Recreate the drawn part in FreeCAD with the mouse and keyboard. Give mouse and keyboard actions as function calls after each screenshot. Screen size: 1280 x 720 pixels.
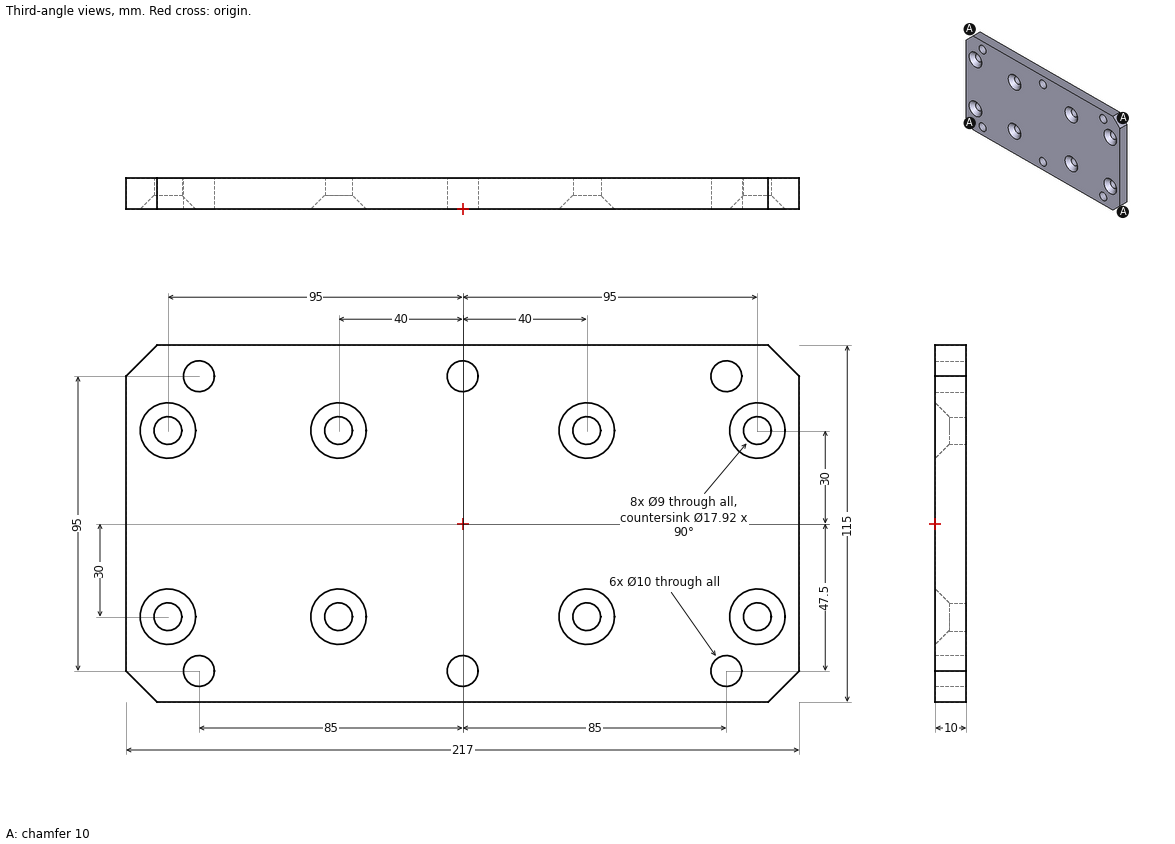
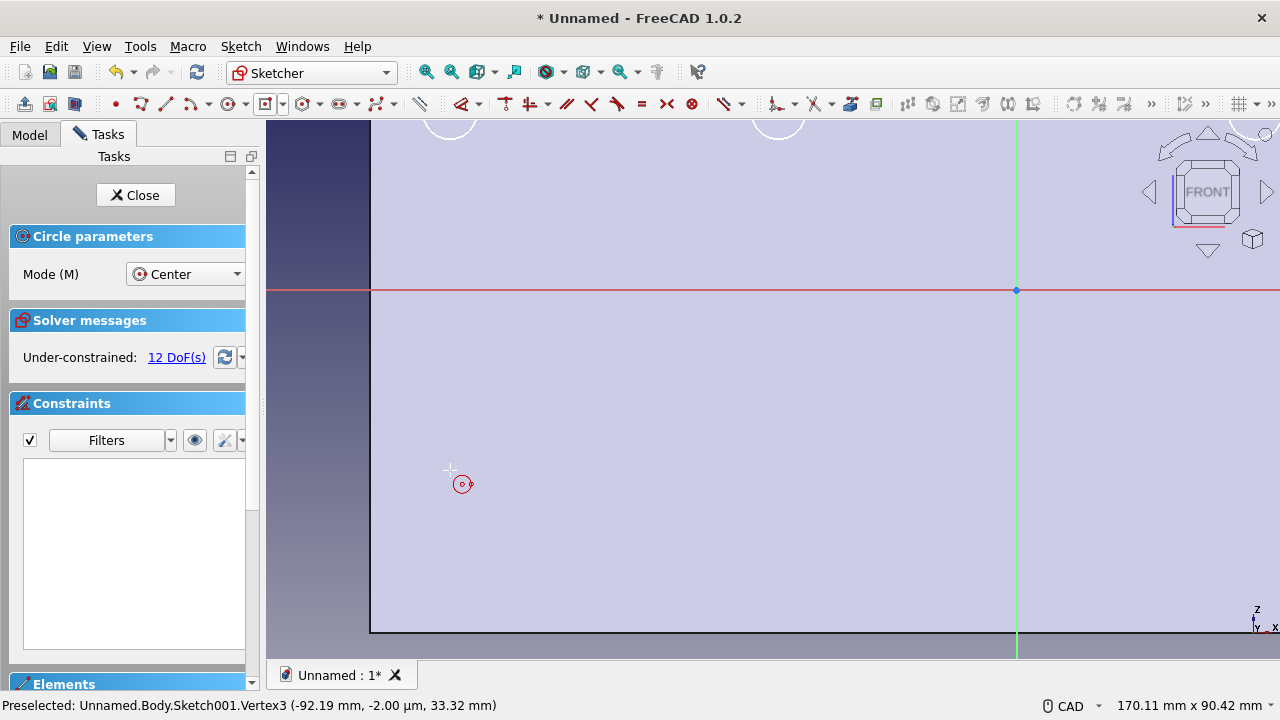
click(450, 469)
click(469, 450)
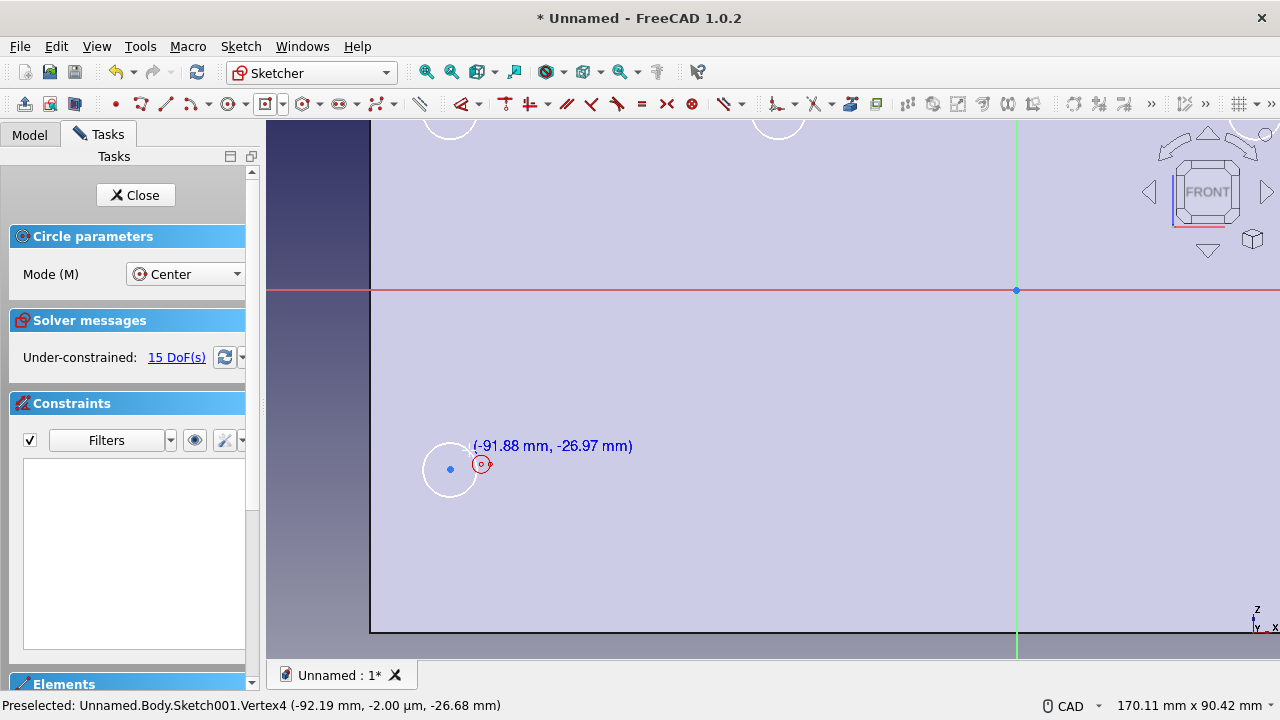
click(778, 469)
click(797, 450)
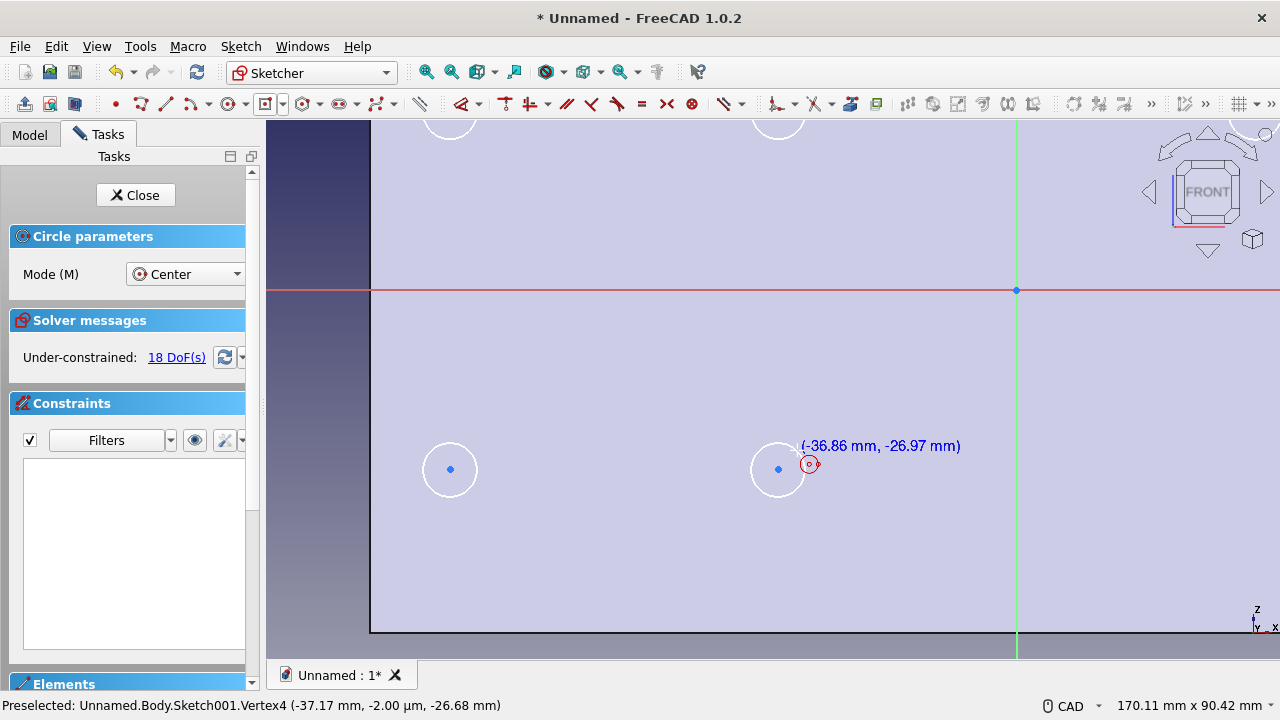
scroll(450, 471, down, 4)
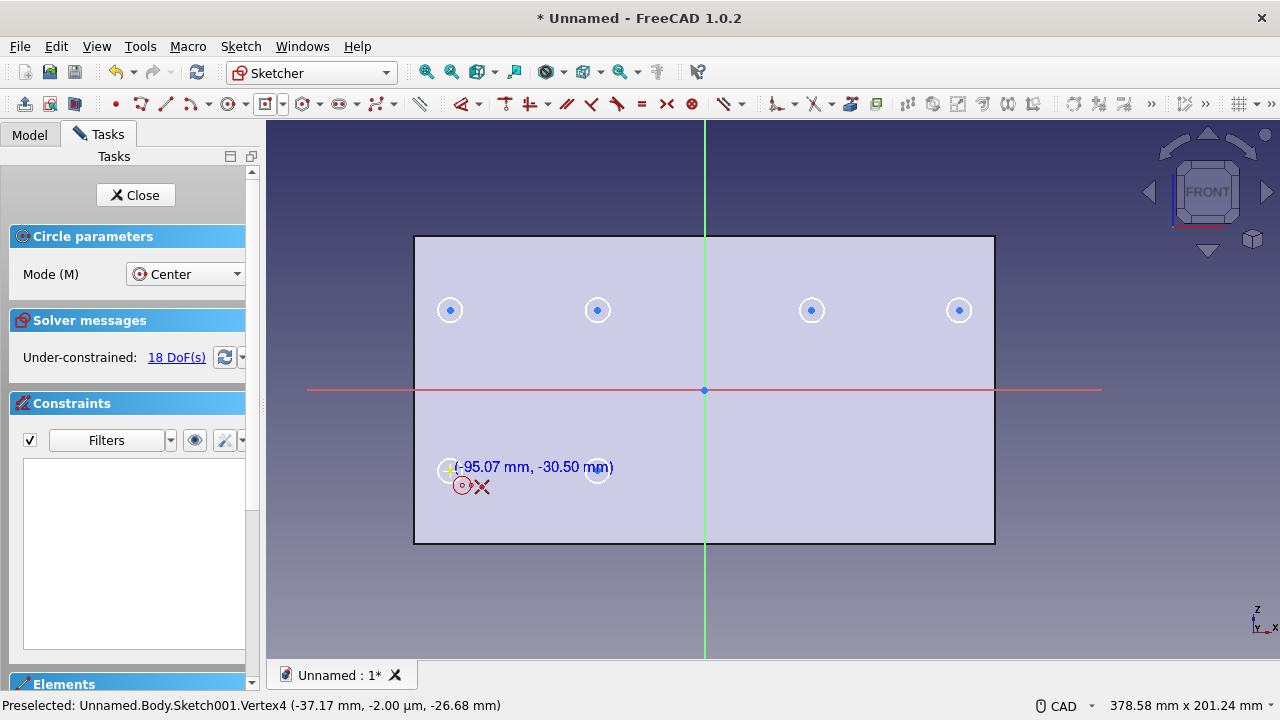
scroll(812, 470, up, 4)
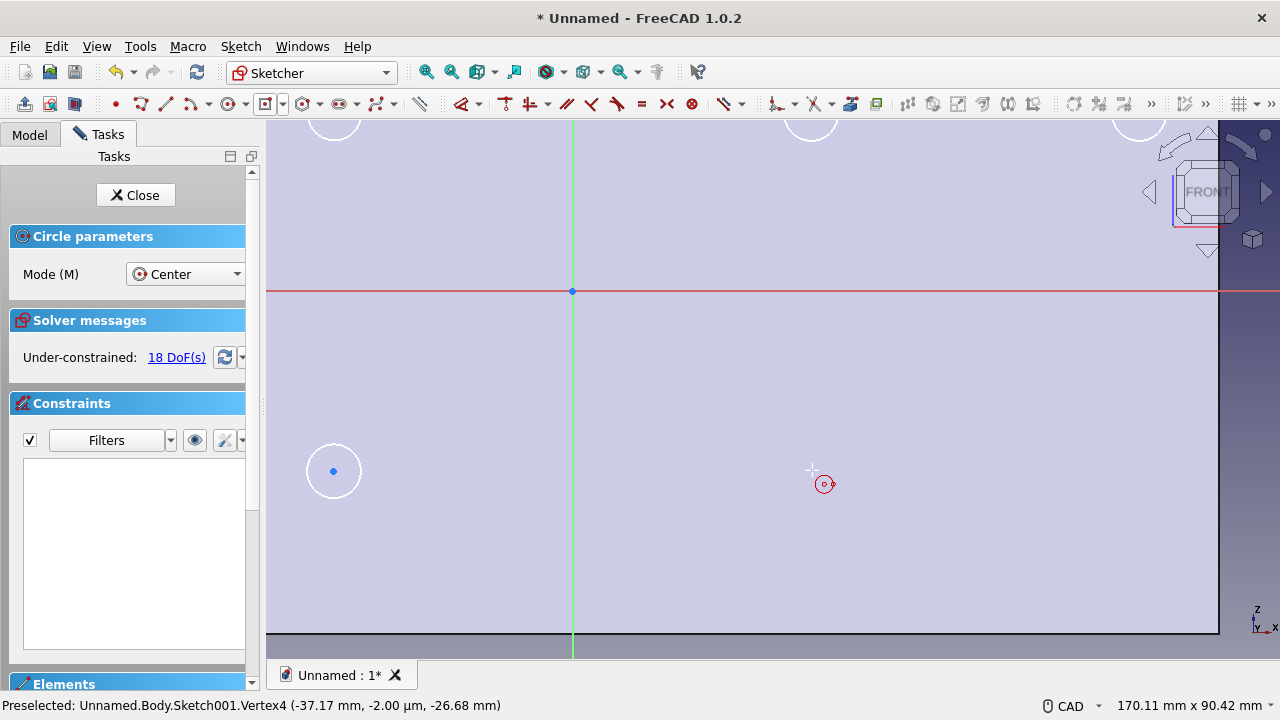
click(811, 470)
click(830, 451)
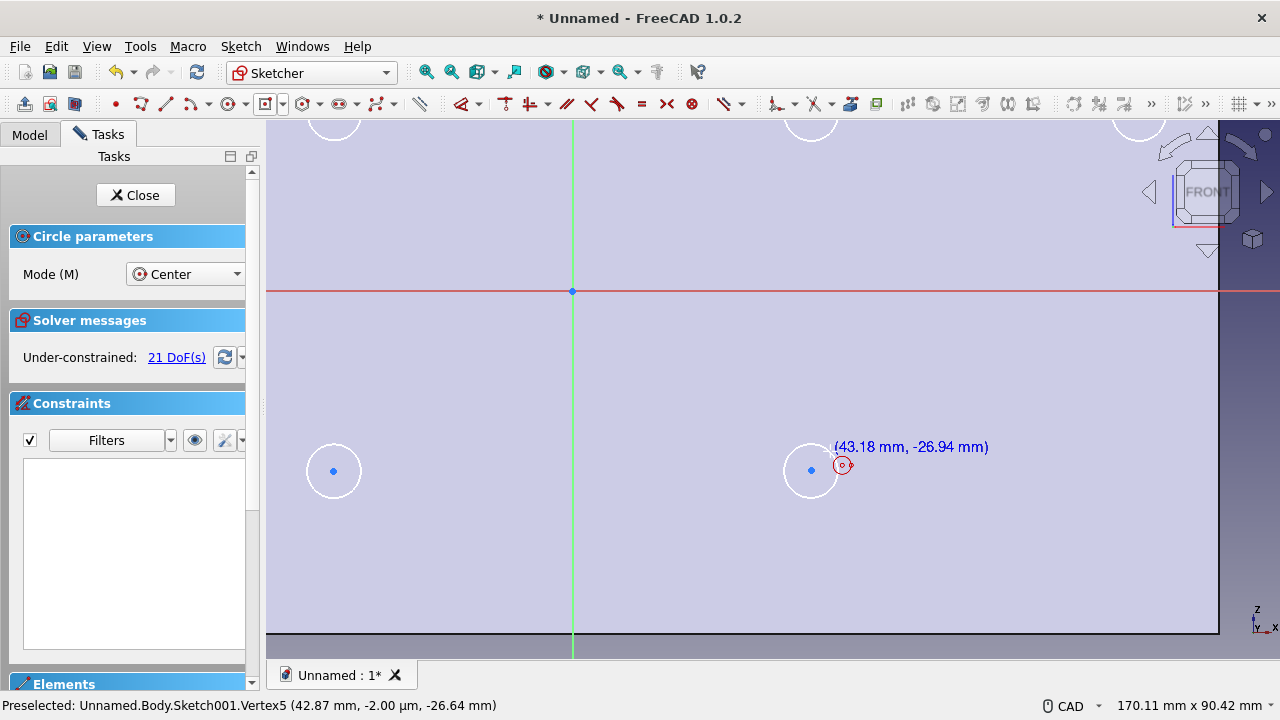
scroll(812, 470, down, 4)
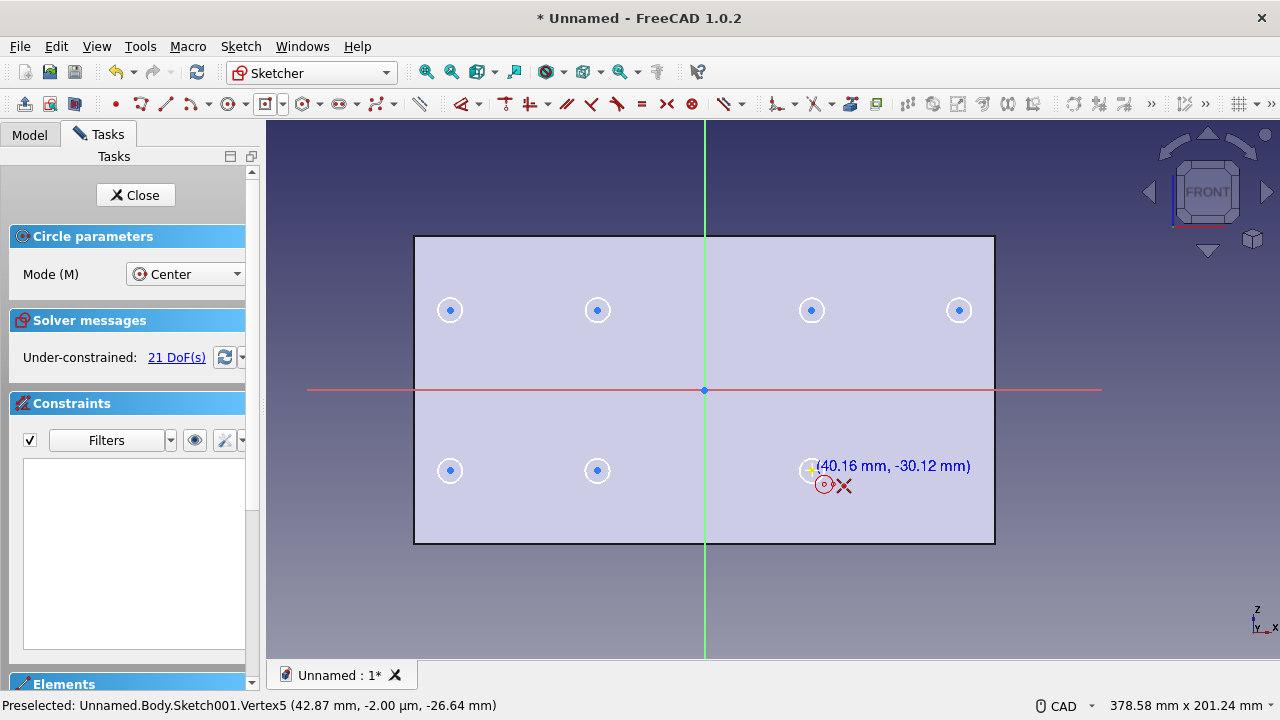
scroll(959, 470, up, 4)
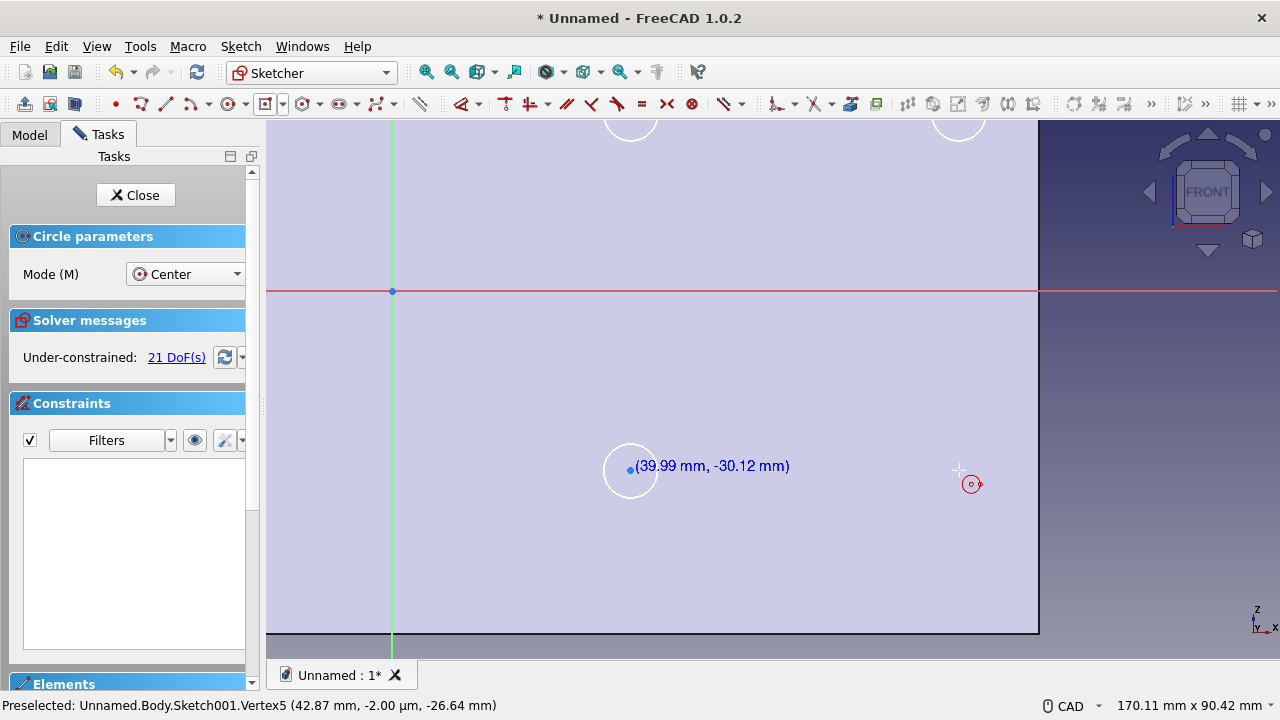
click(959, 470)
click(978, 451)
key(Escape)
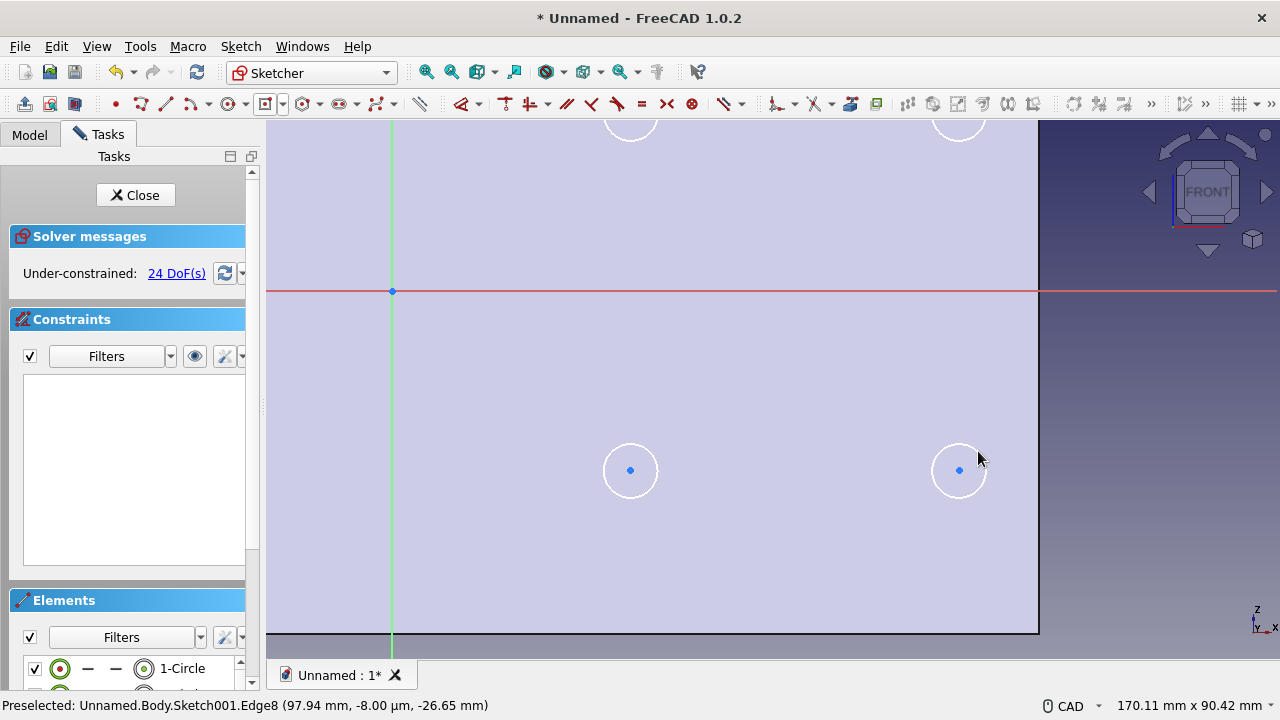
scroll(959, 470, down, 4)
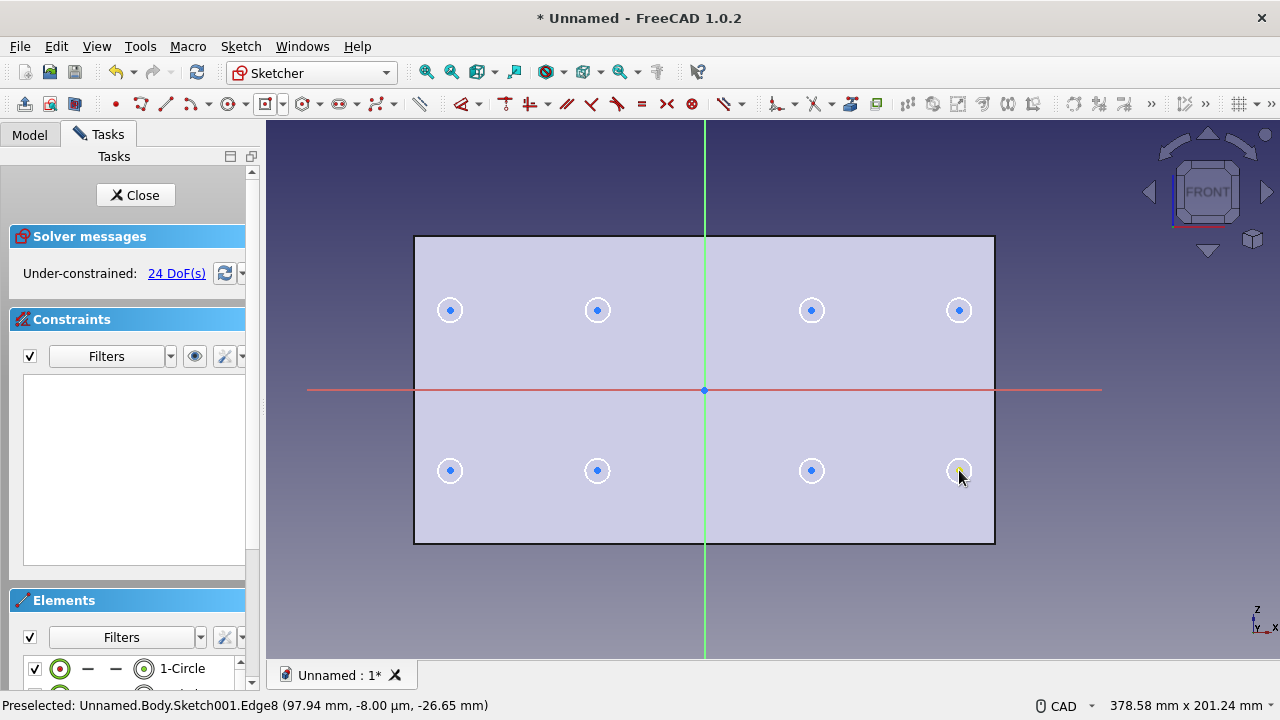
click(968, 302)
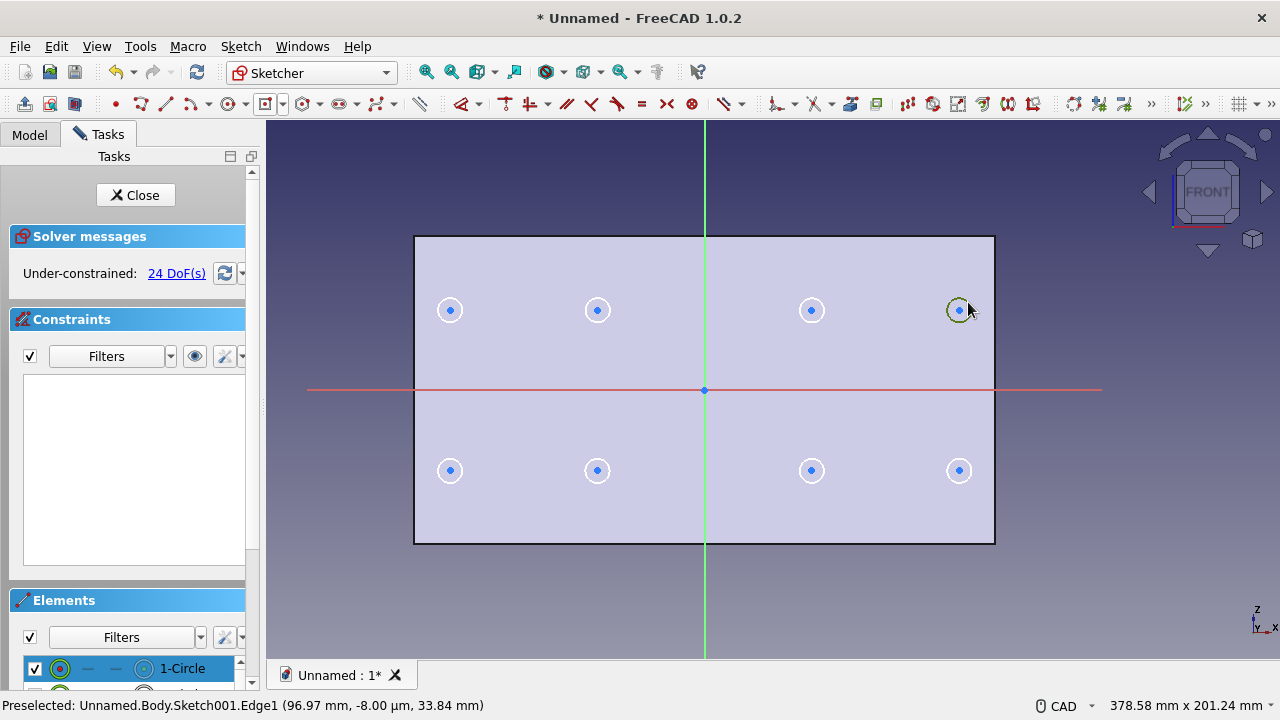
click(820, 302)